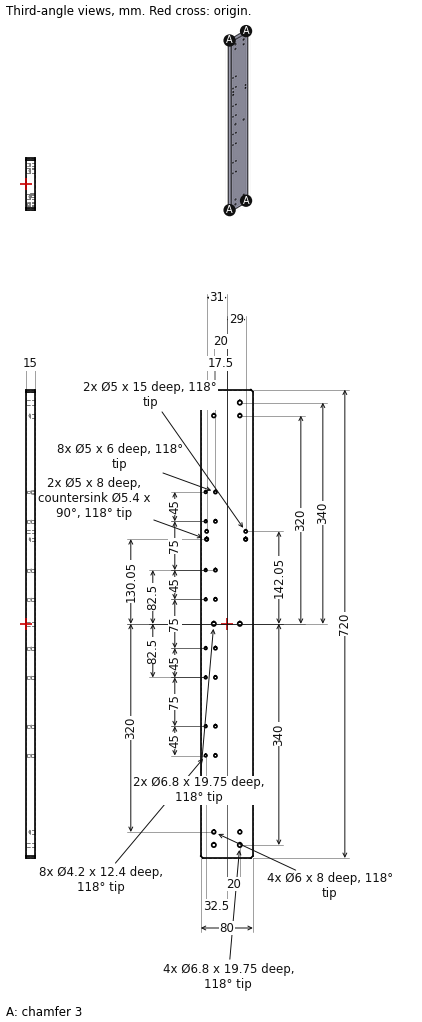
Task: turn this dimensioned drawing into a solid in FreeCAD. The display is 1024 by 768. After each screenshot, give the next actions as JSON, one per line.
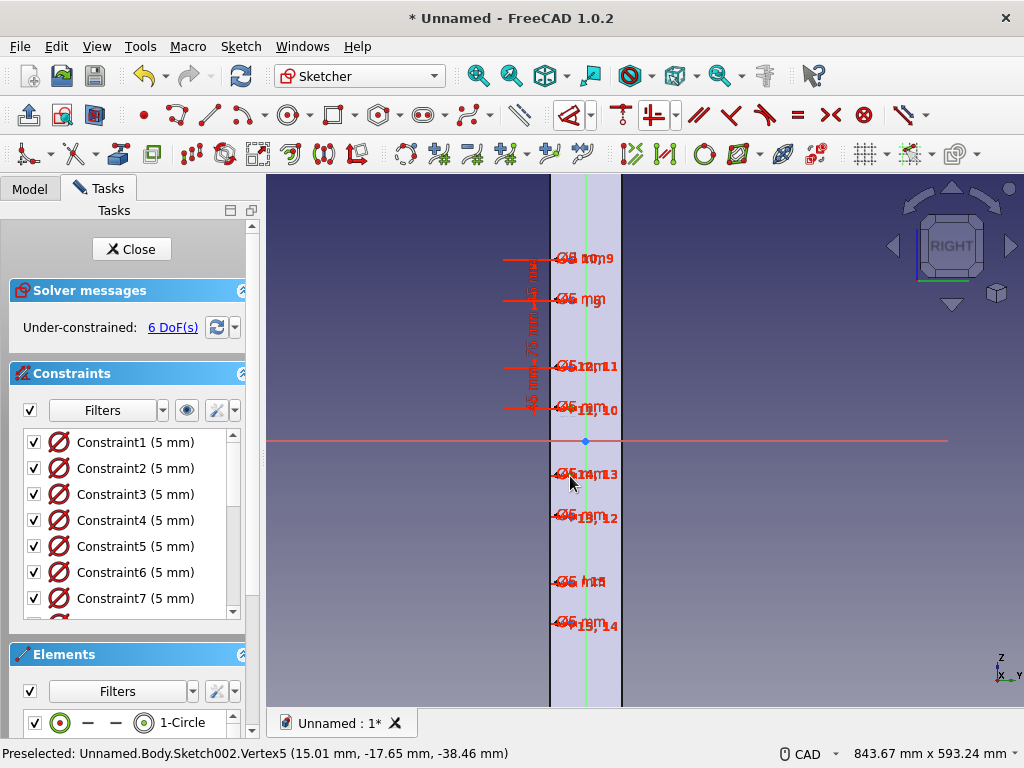
{"action": "key", "text": "i"}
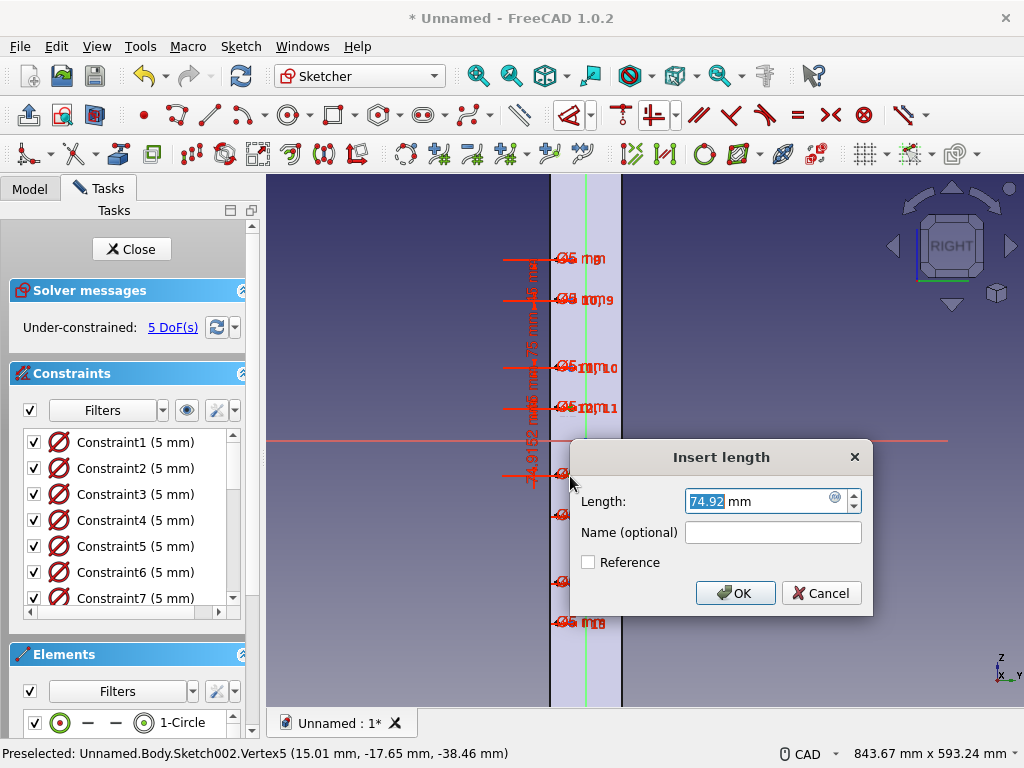
{"action": "type", "text": "75"}
{"action": "key", "text": "Return"}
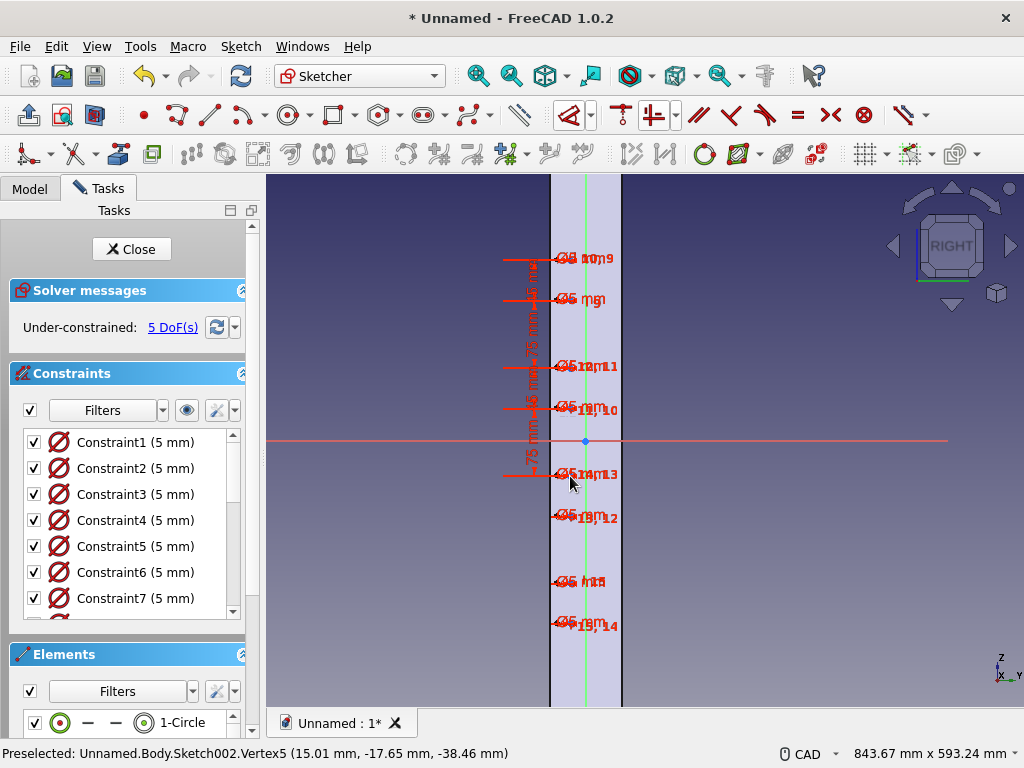
{"action": "left_click", "coordinate": [570, 476]}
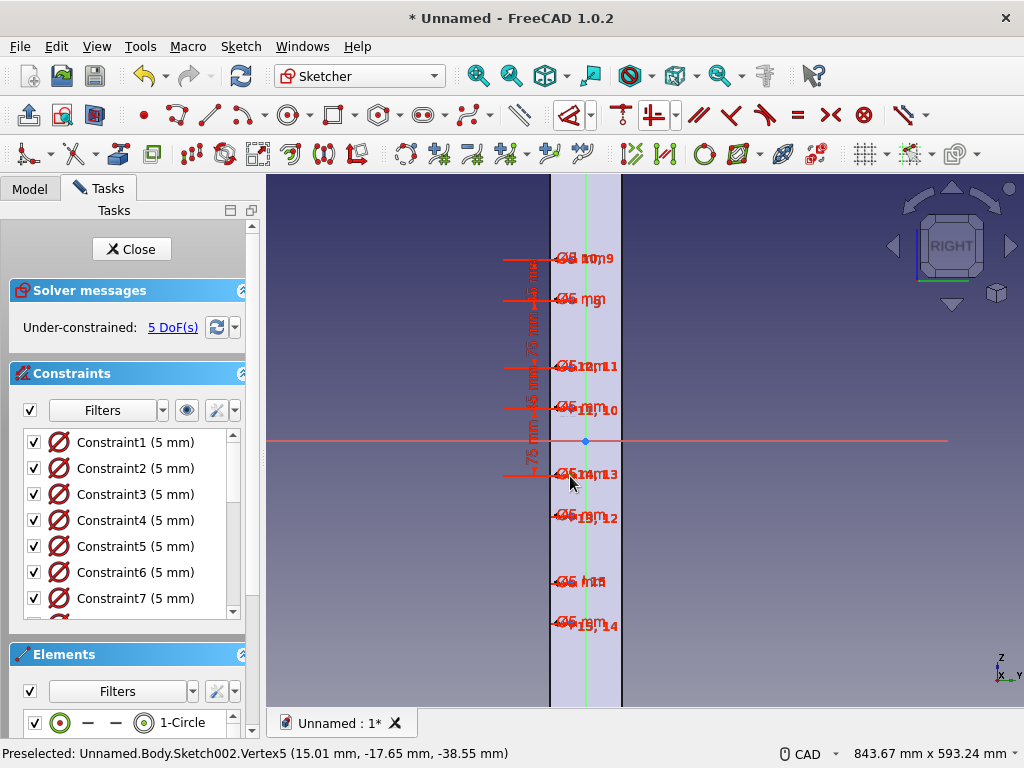
{"action": "left_click", "coordinate": [570, 517]}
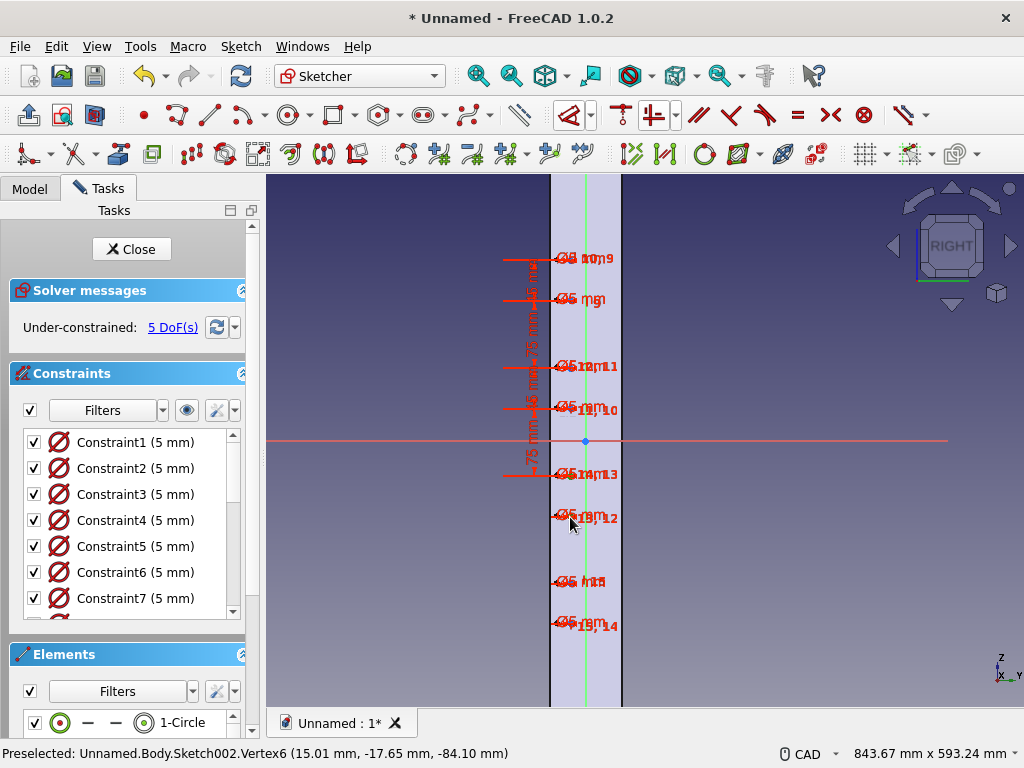
{"action": "key", "text": "i"}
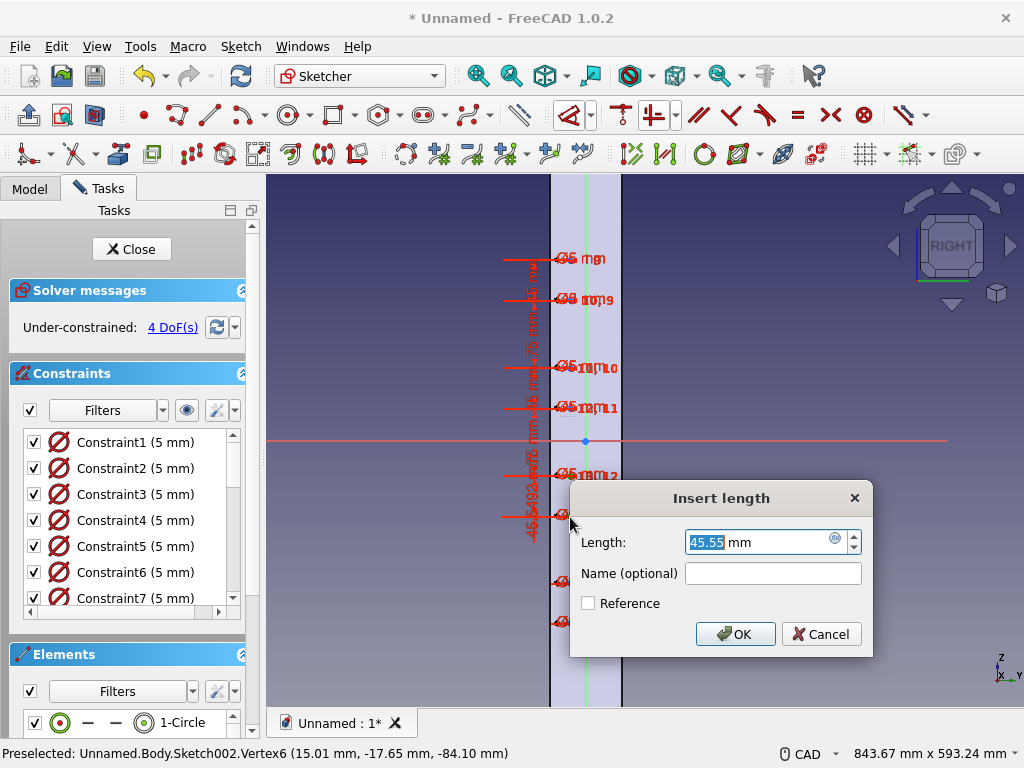
{"action": "type", "text": "45"}
{"action": "key", "text": "Return"}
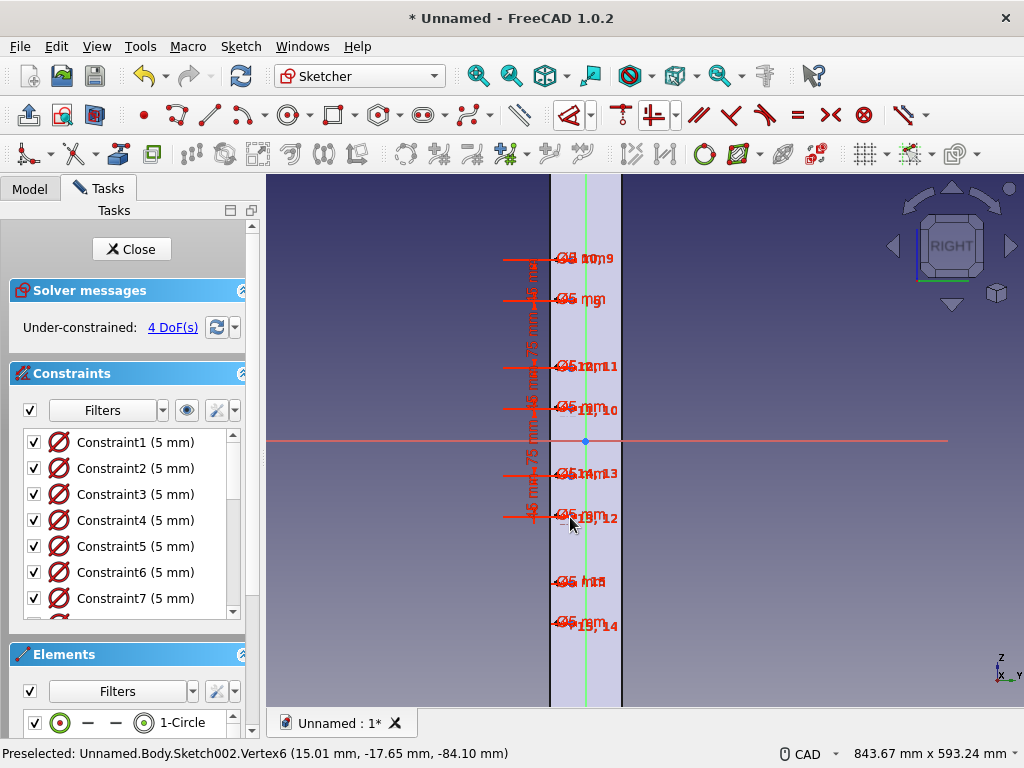
{"action": "left_click", "coordinate": [570, 517]}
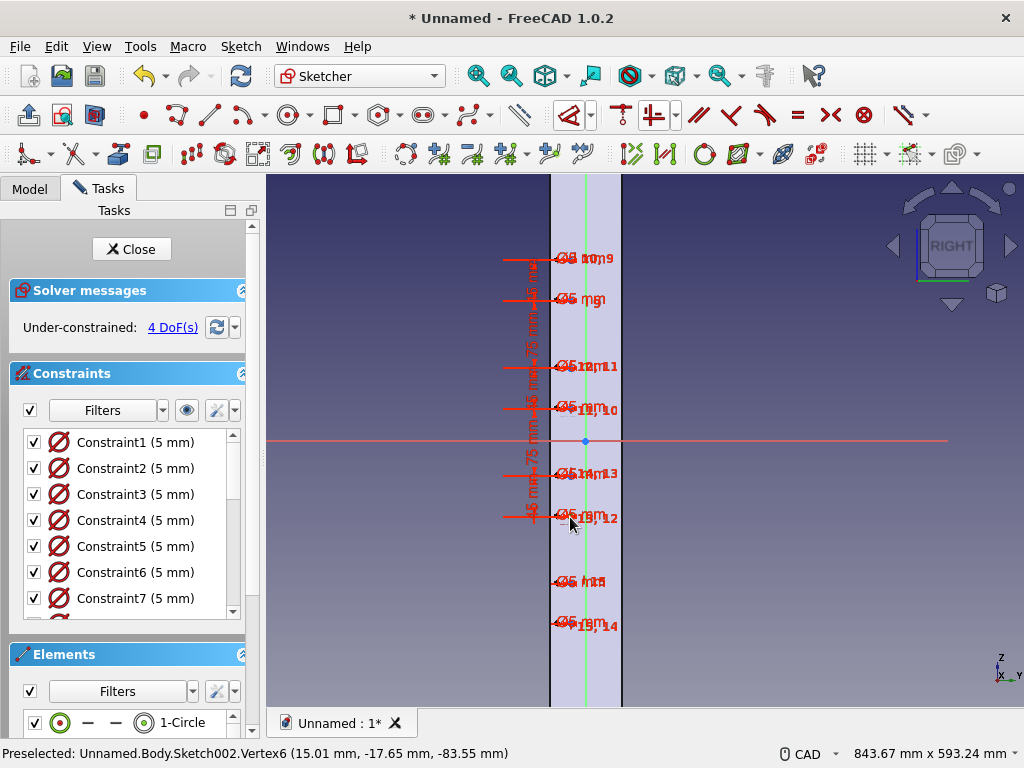
{"action": "left_click", "coordinate": [570, 584]}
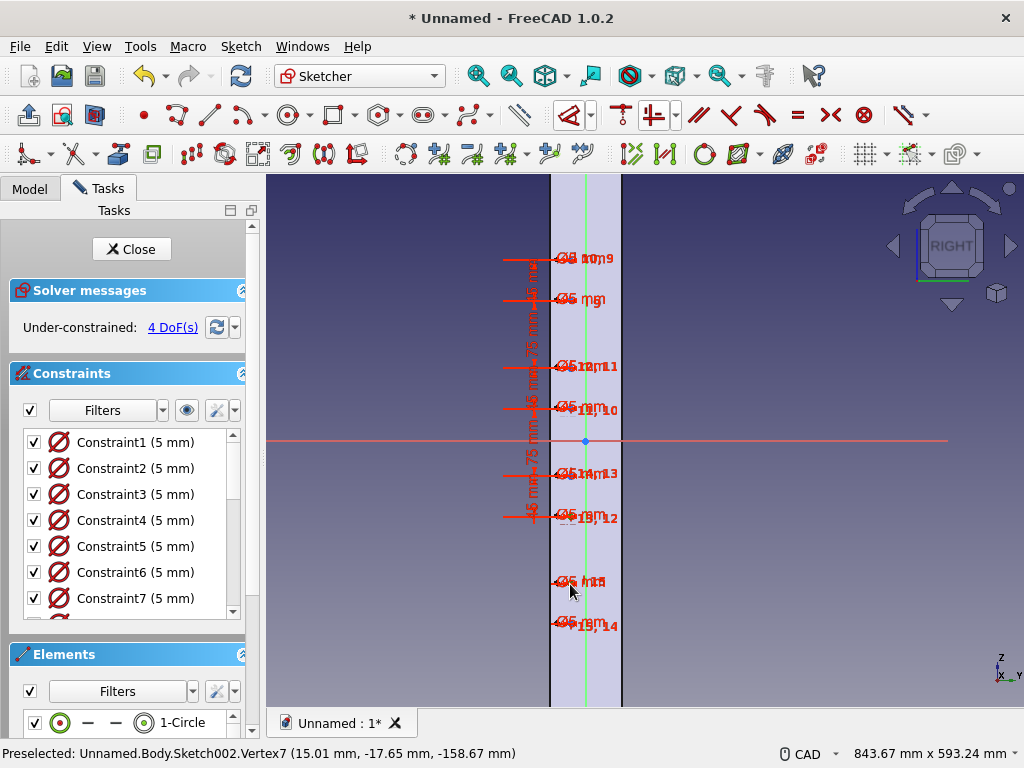
{"action": "left_click", "coordinate": [590, 116]}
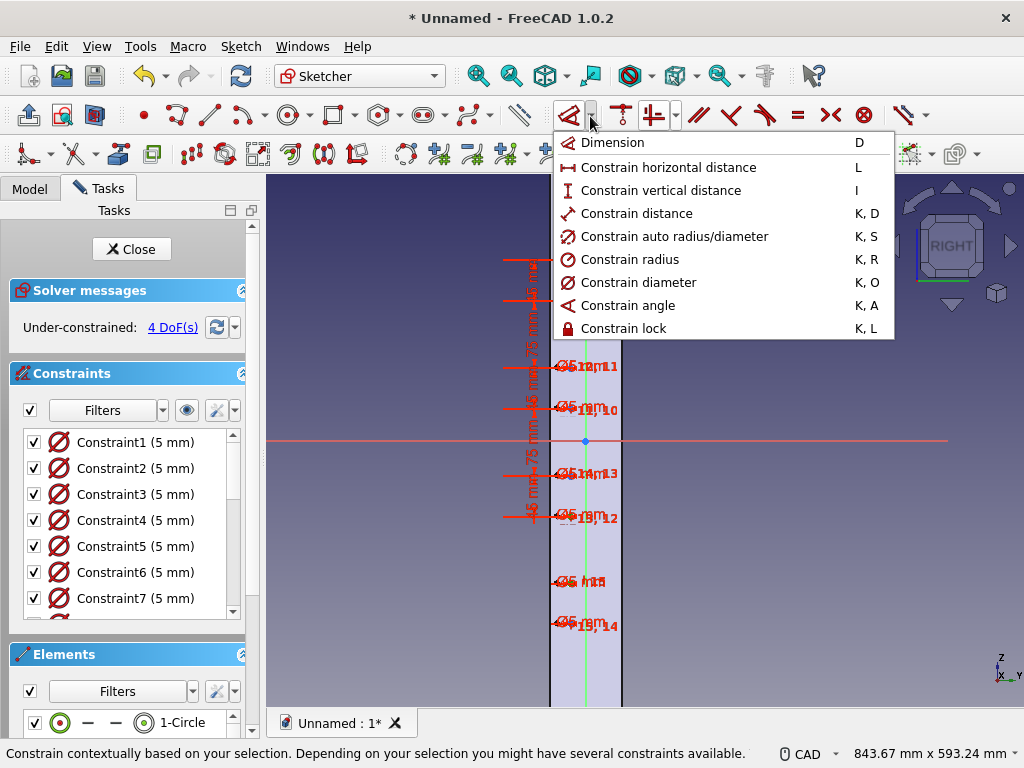
{"action": "left_click", "coordinate": [724, 190]}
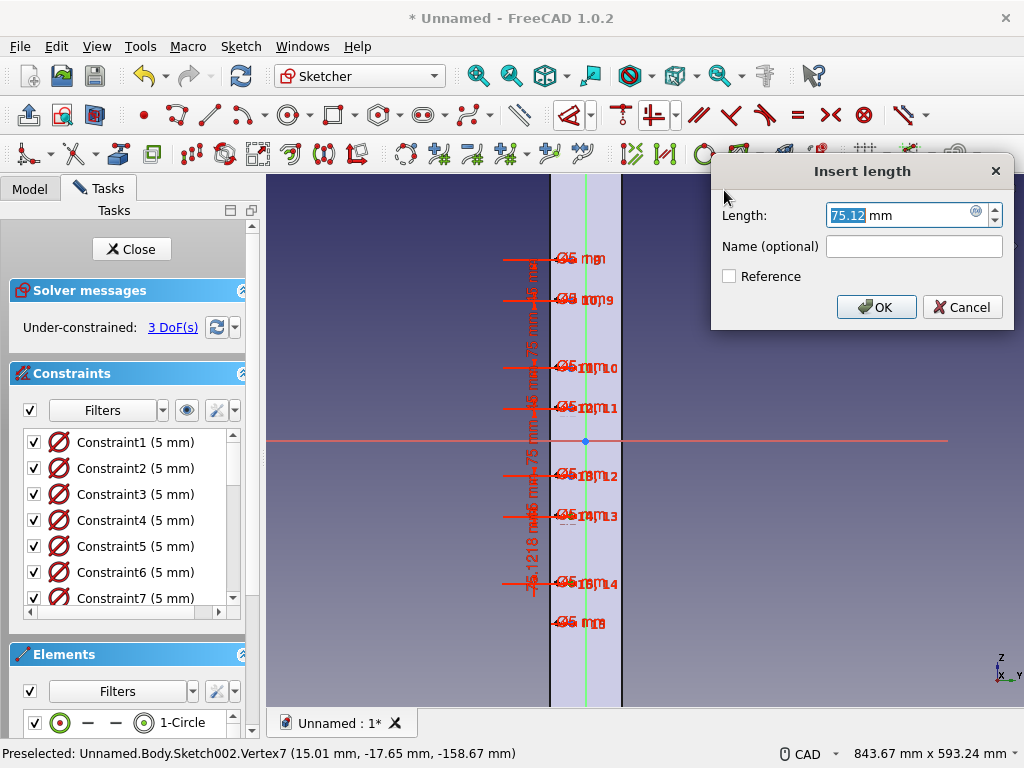
{"action": "type", "text": "75"}
{"action": "key", "text": "Return"}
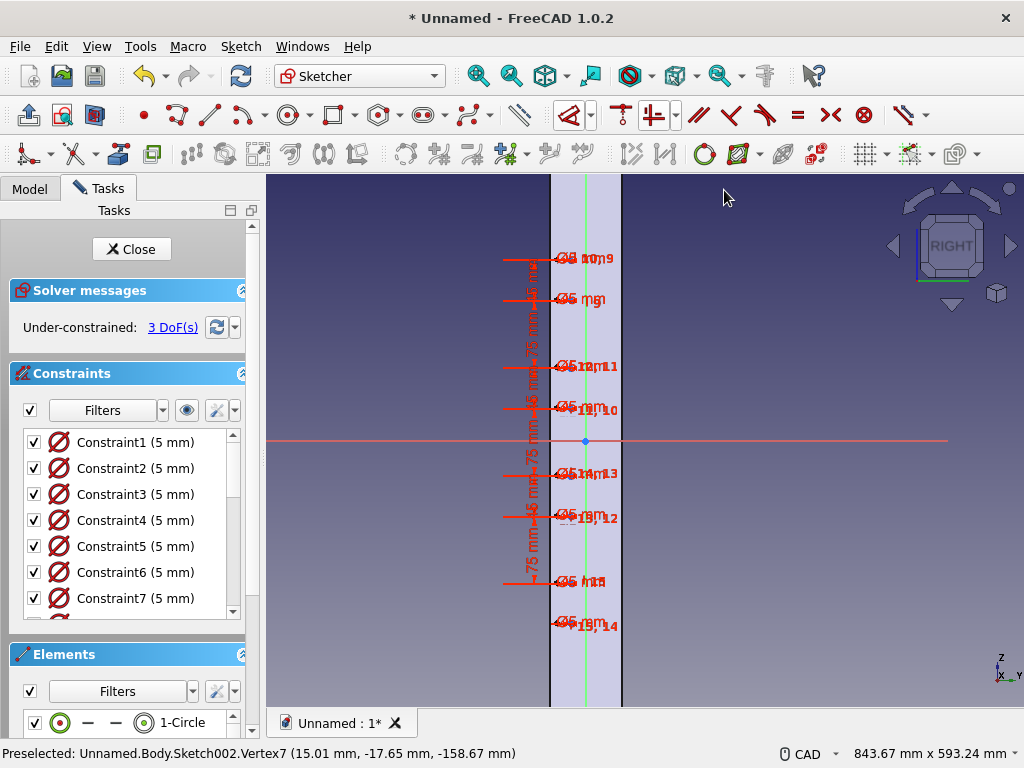
{"action": "left_click", "coordinate": [570, 584]}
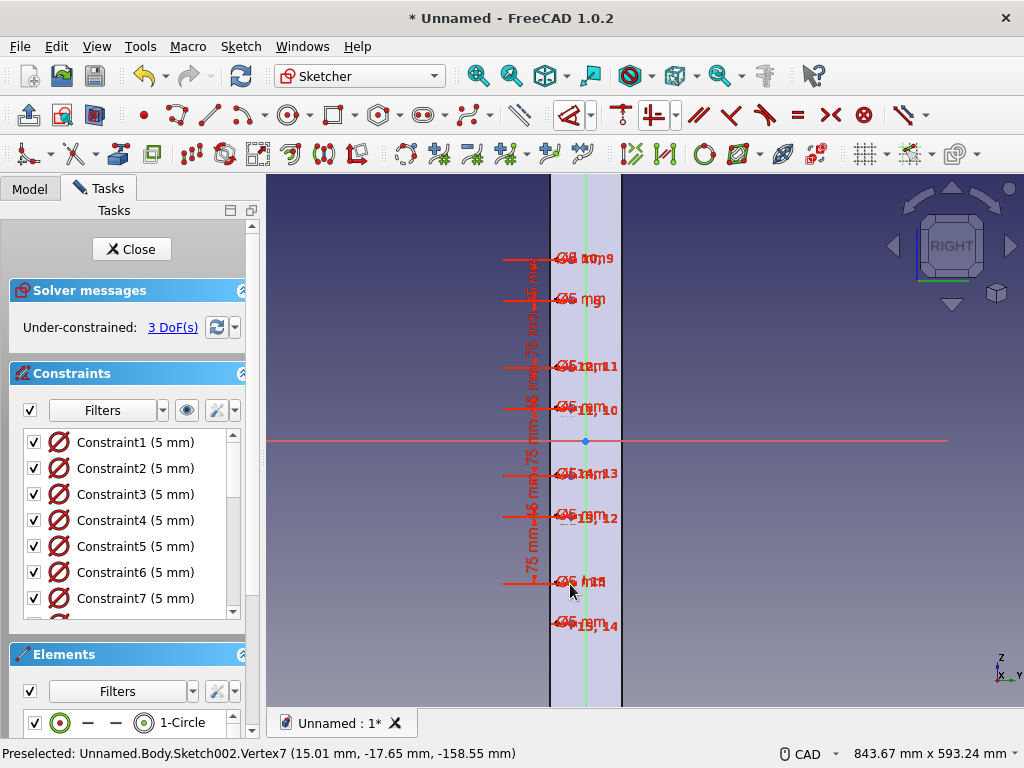
{"action": "left_click", "coordinate": [570, 624]}